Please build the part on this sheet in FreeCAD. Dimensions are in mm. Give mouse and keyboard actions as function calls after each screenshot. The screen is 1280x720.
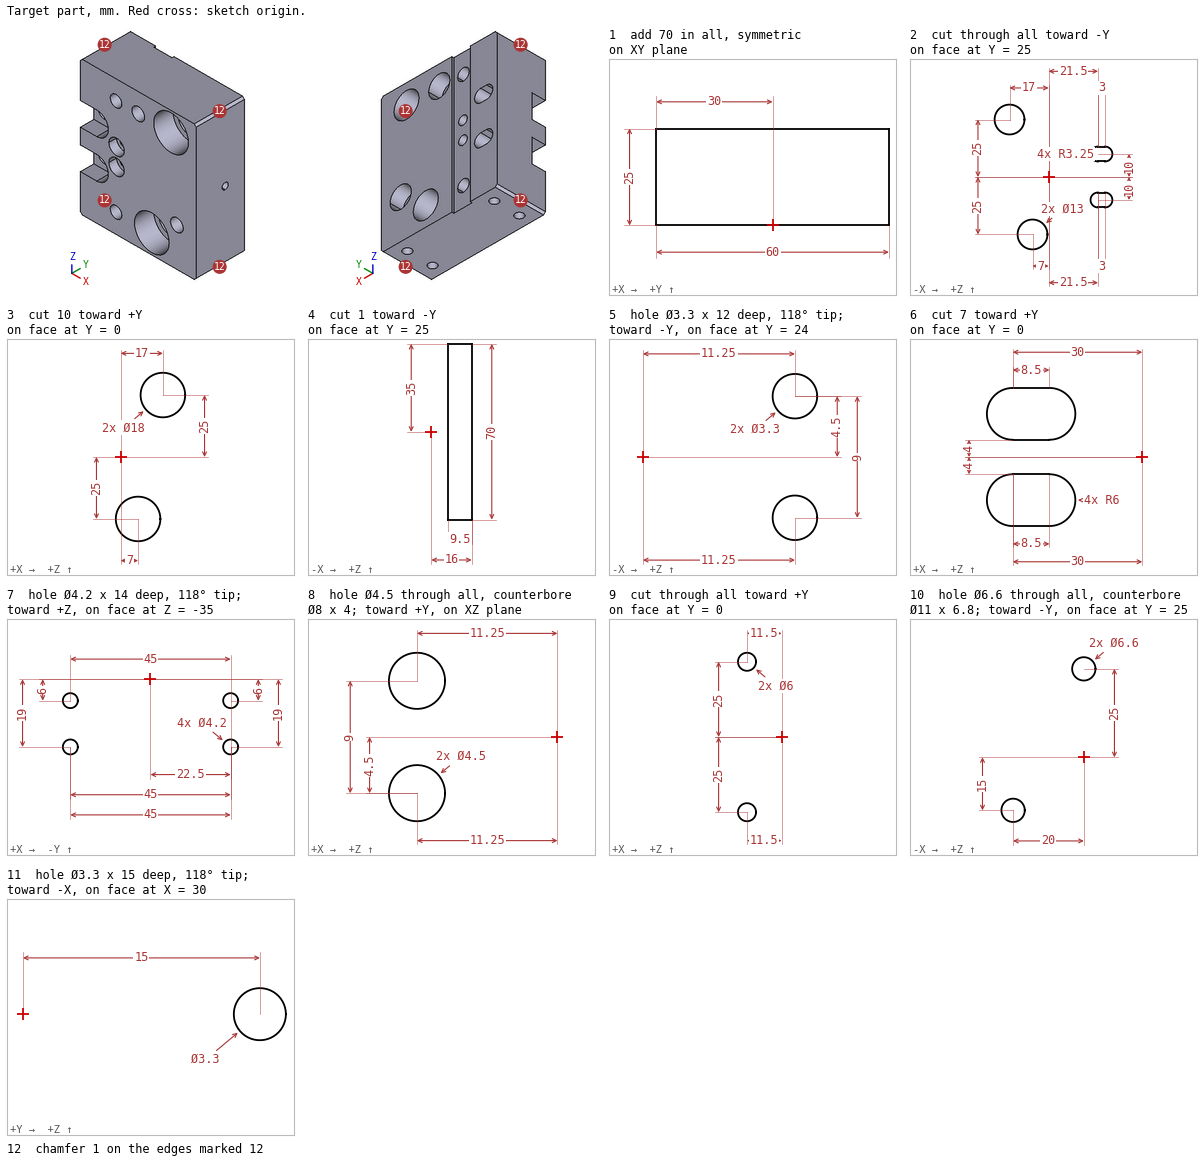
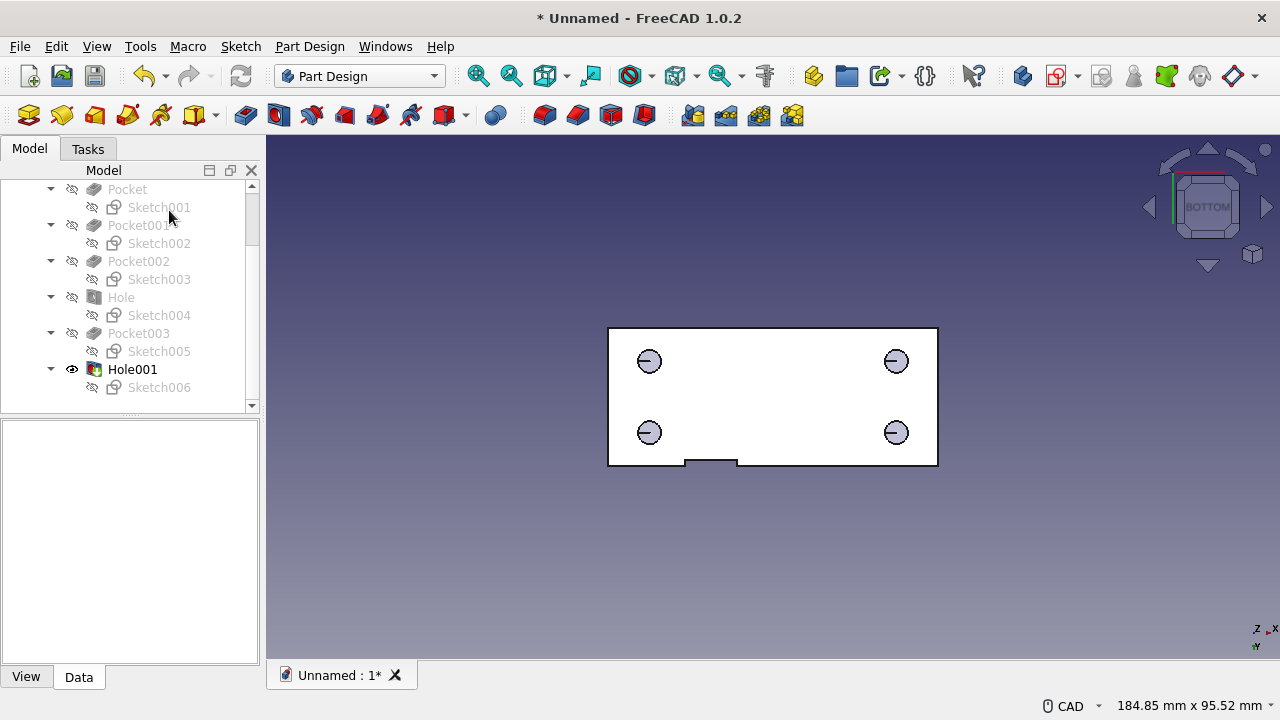
click(1056, 76)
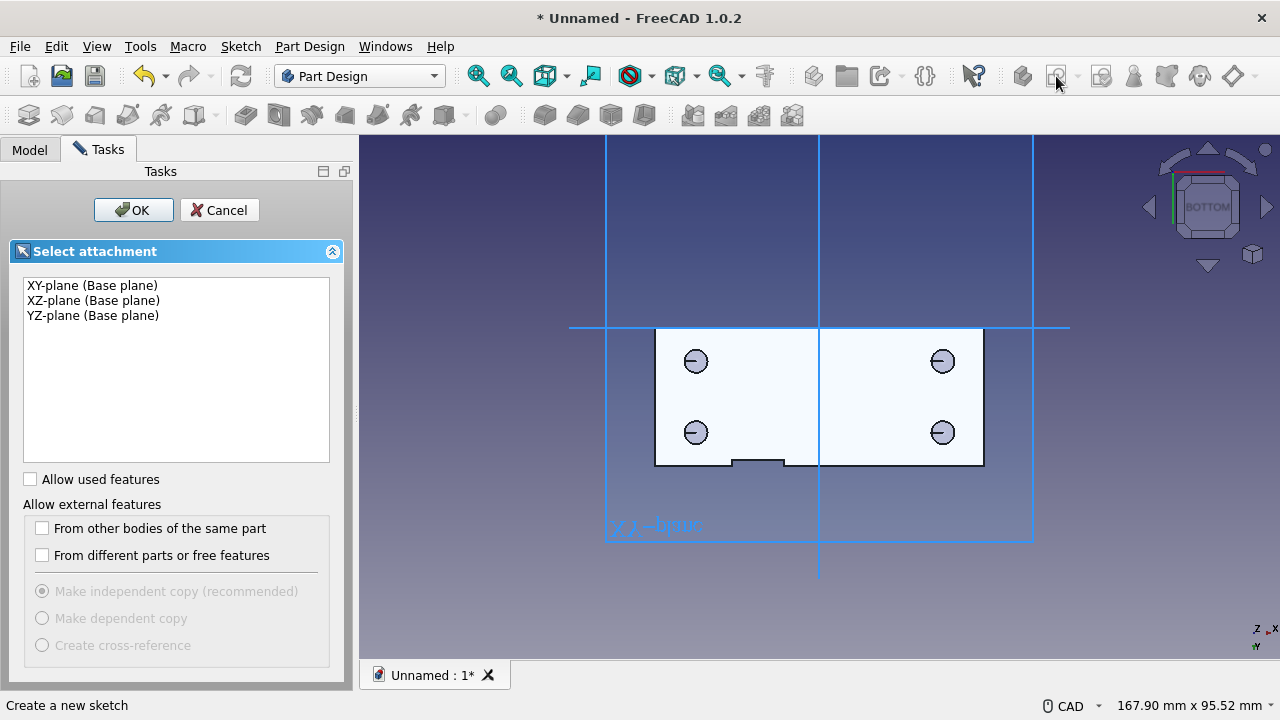
click(84, 300)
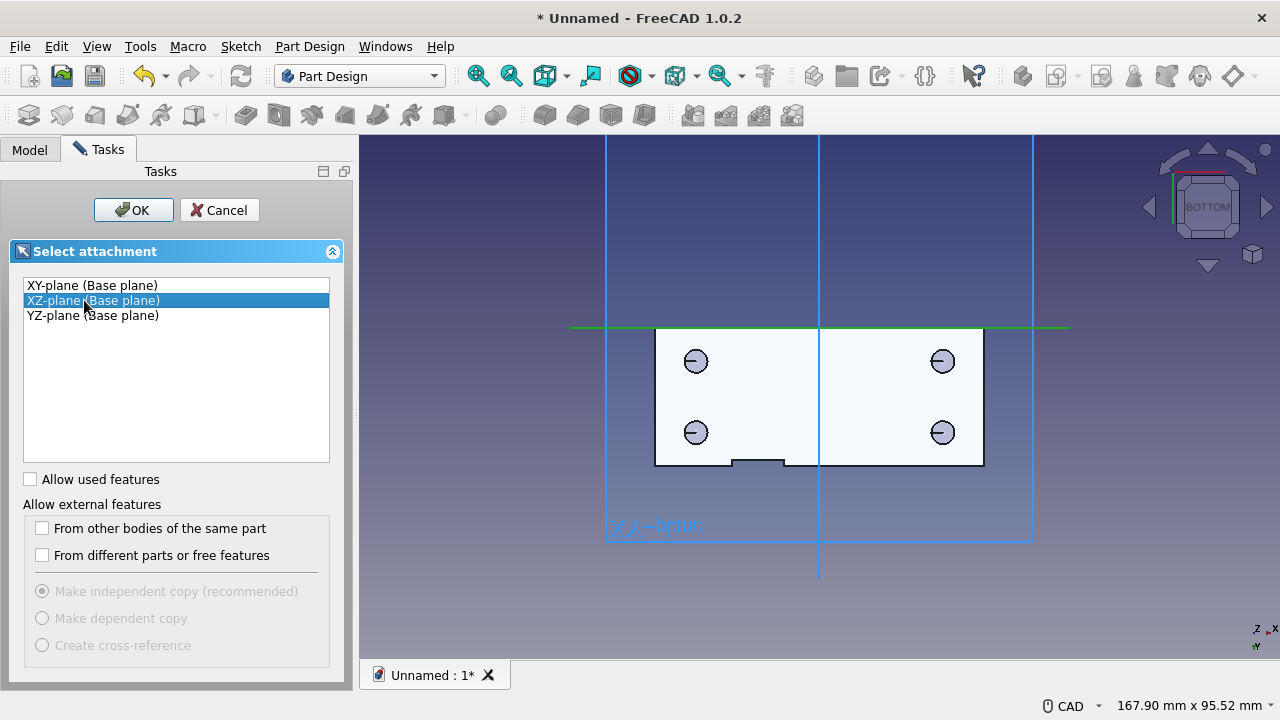
click(134, 210)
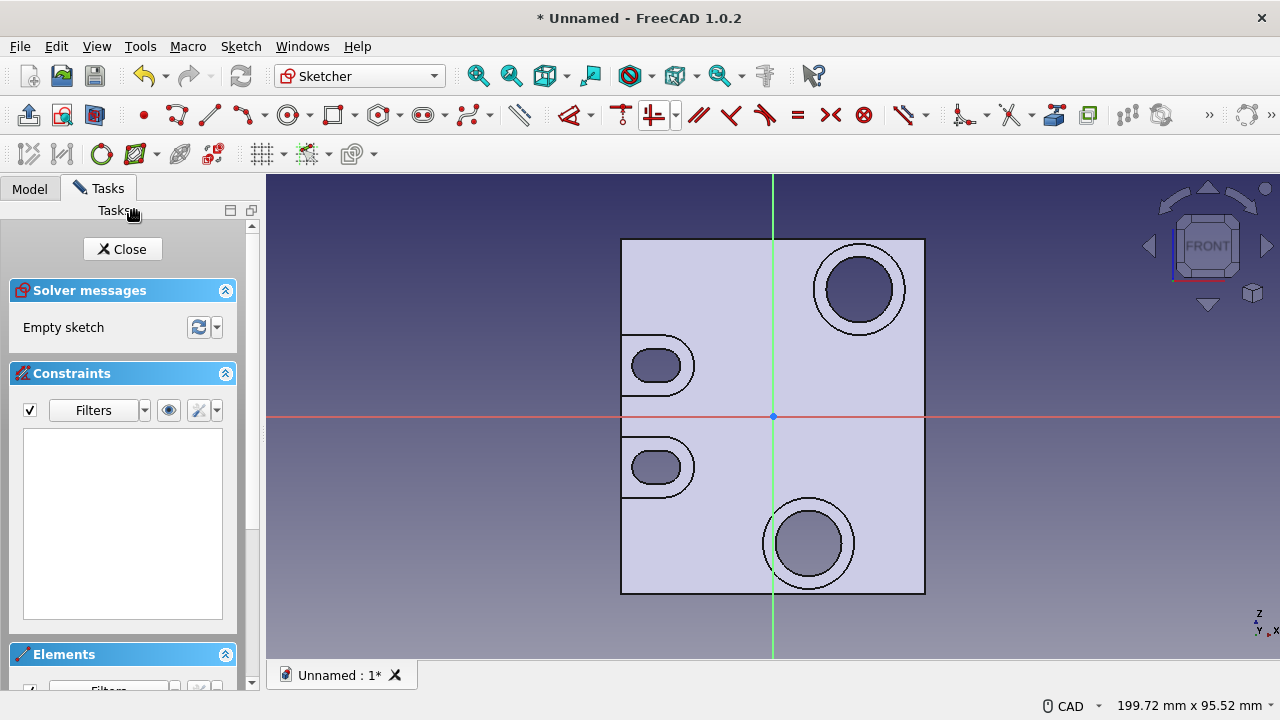
scroll(750, 416, up, 7)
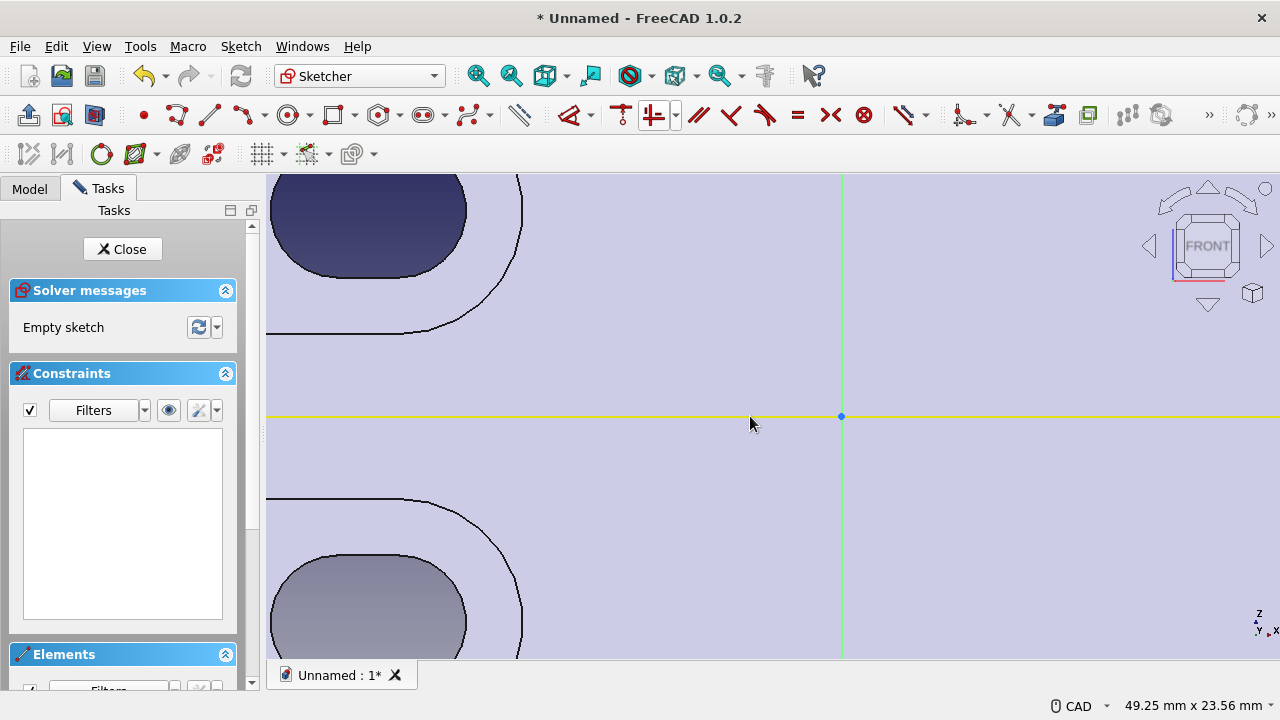
click(288, 116)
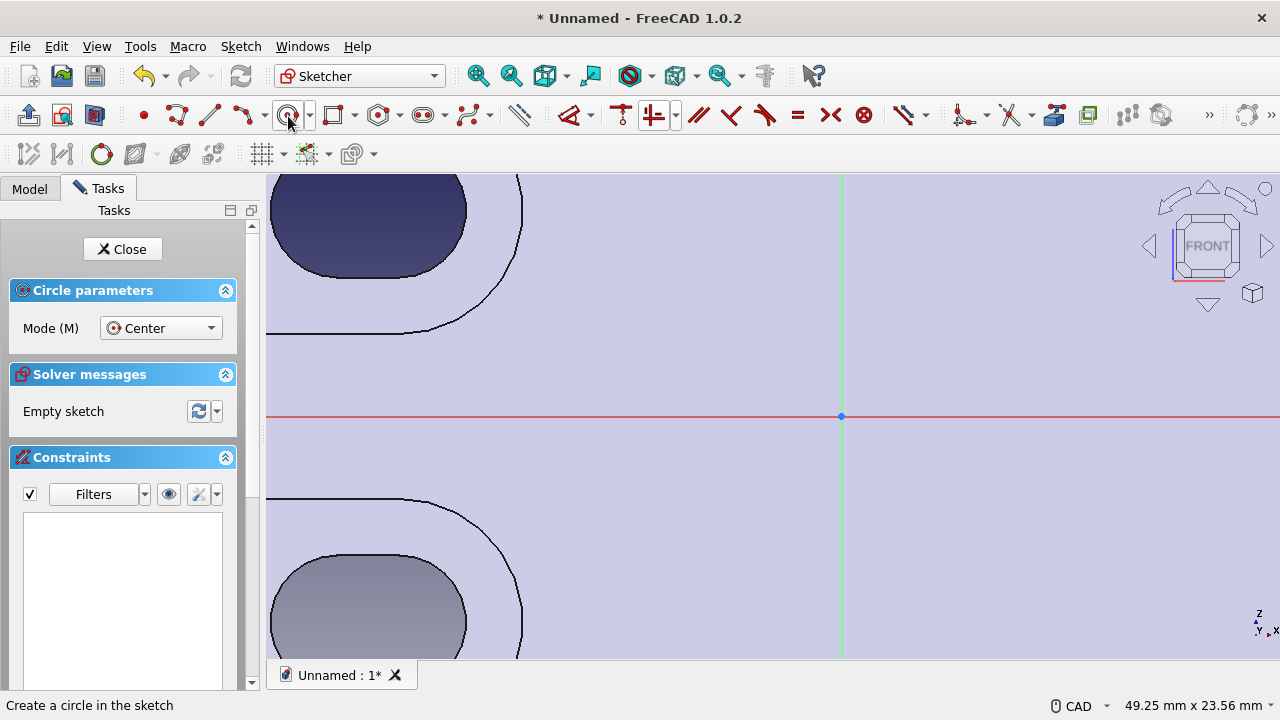
click(610, 509)
move(643, 476)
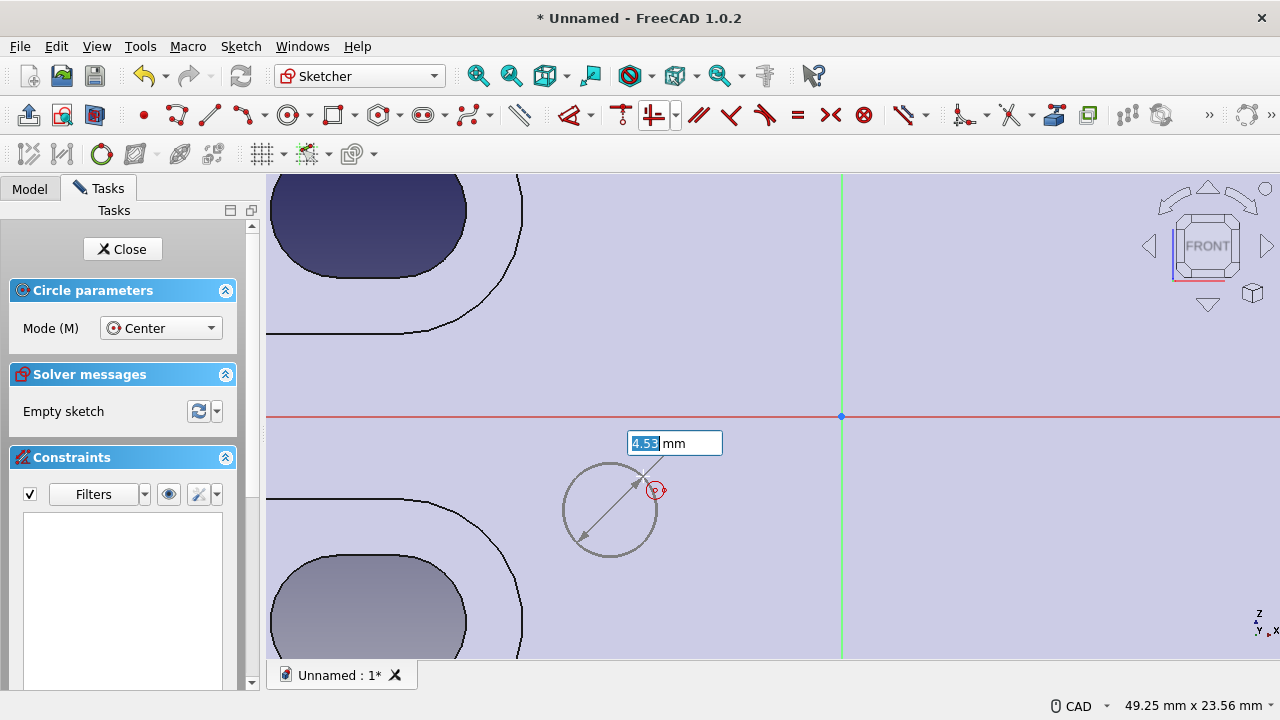
text(4.5)
key(Return)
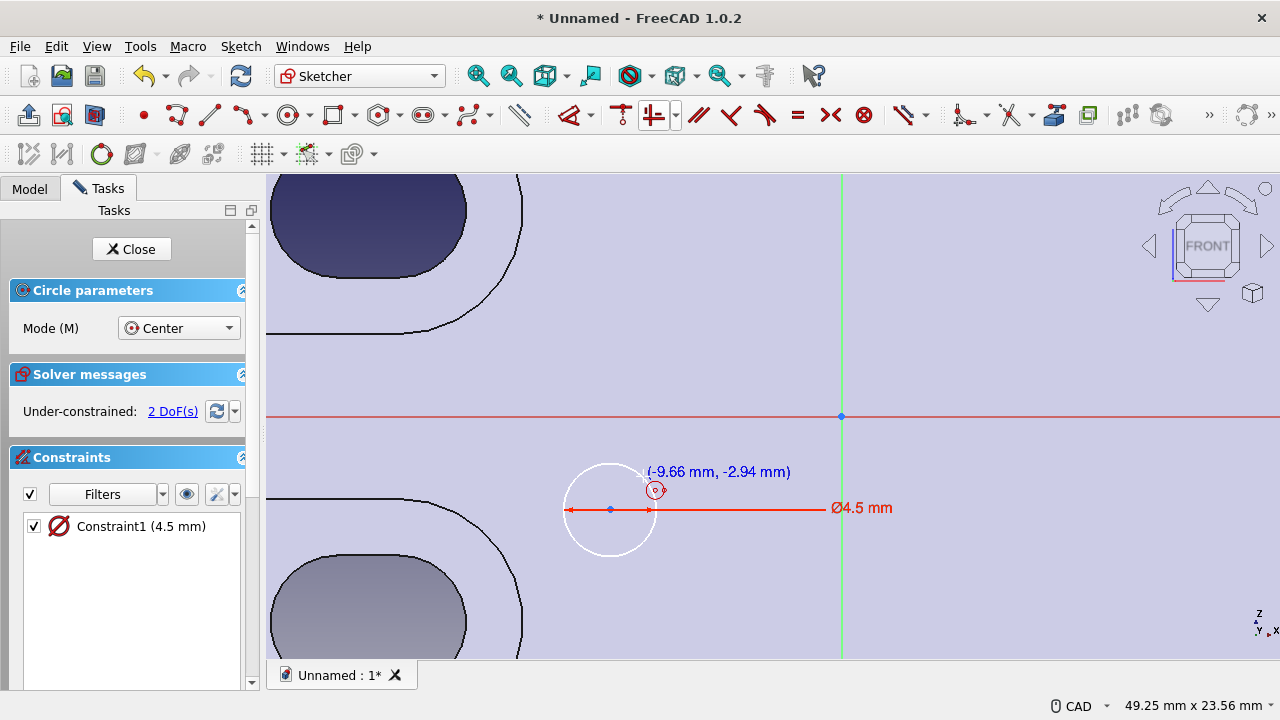
click(610, 324)
move(643, 291)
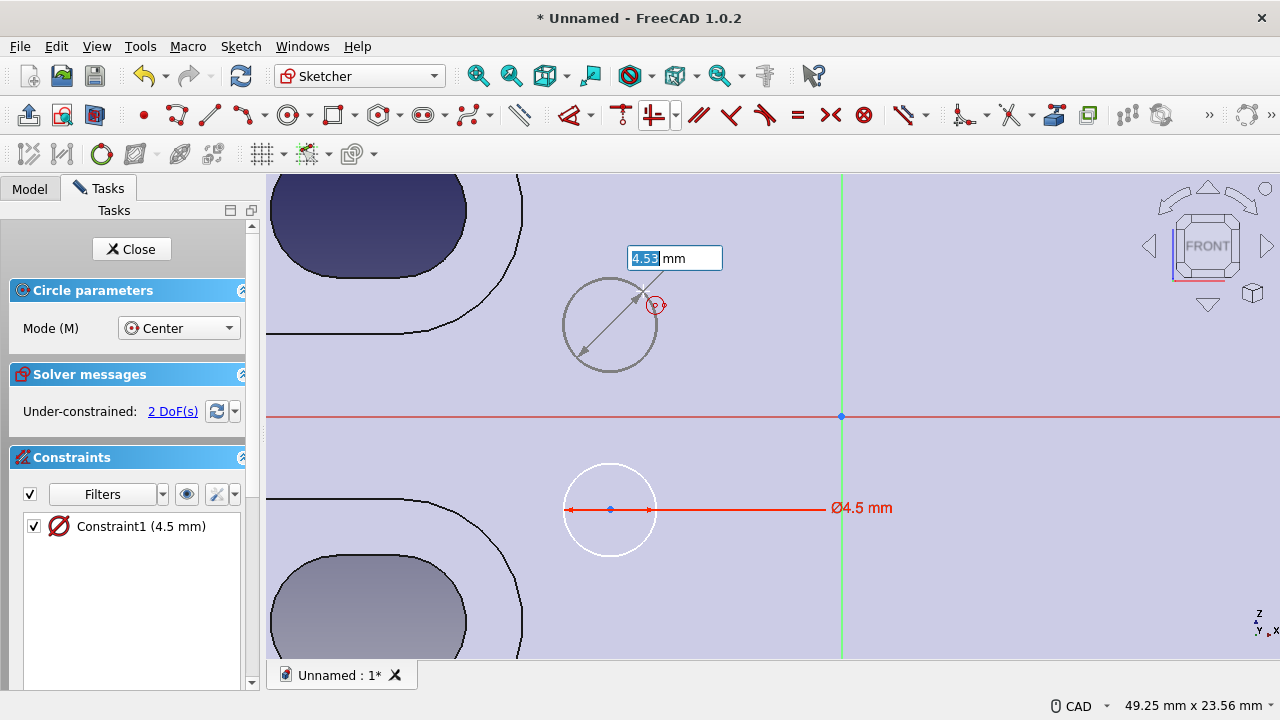
text(4.5)
key(Return)
key(Escape)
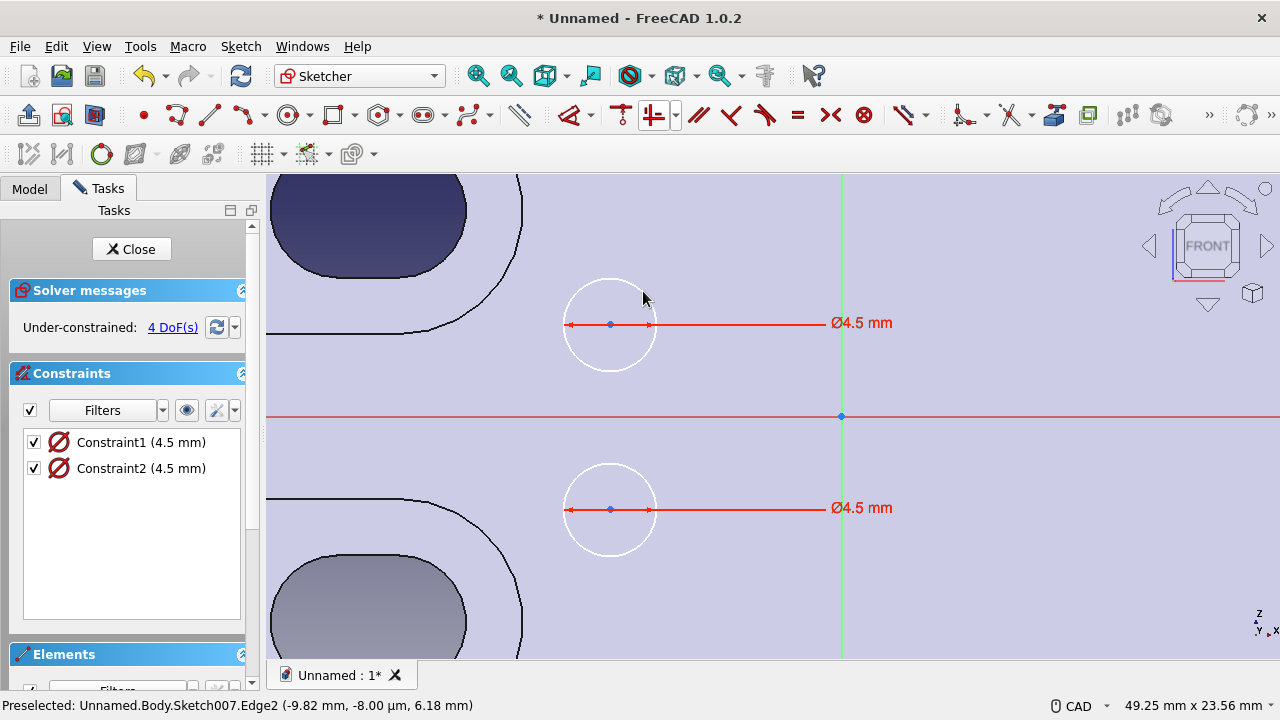
click(568, 116)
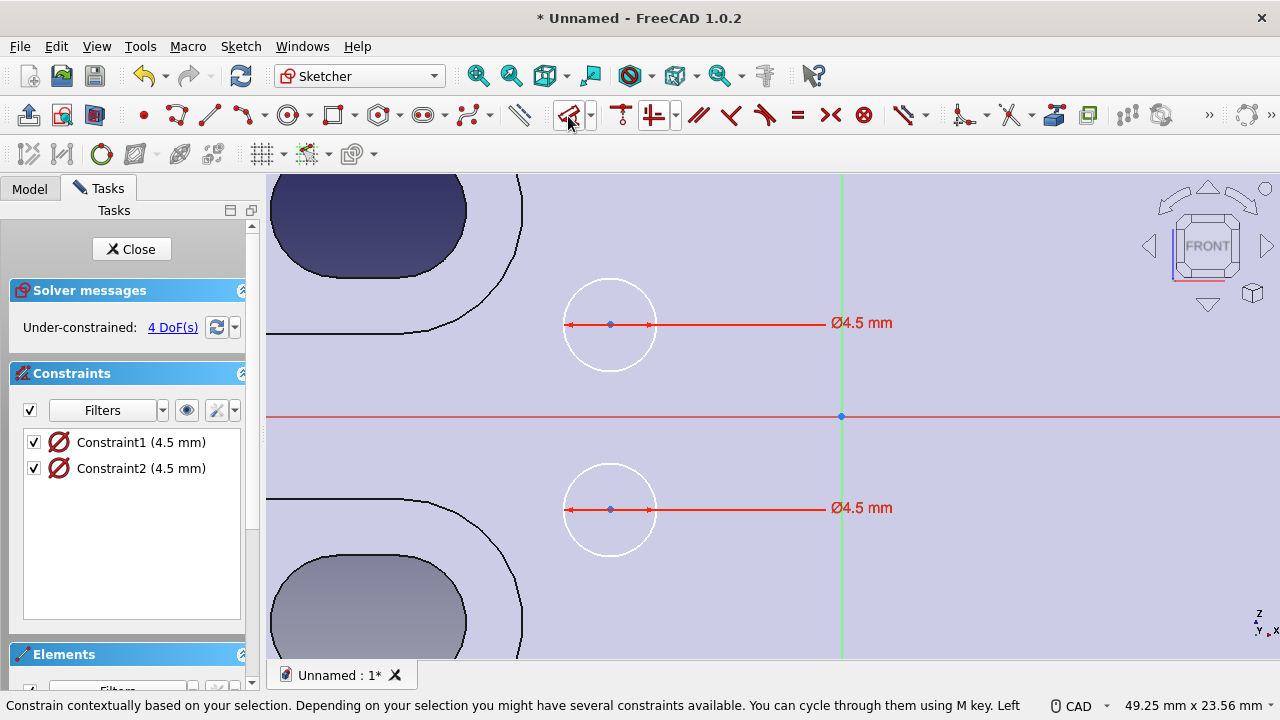
click(610, 510)